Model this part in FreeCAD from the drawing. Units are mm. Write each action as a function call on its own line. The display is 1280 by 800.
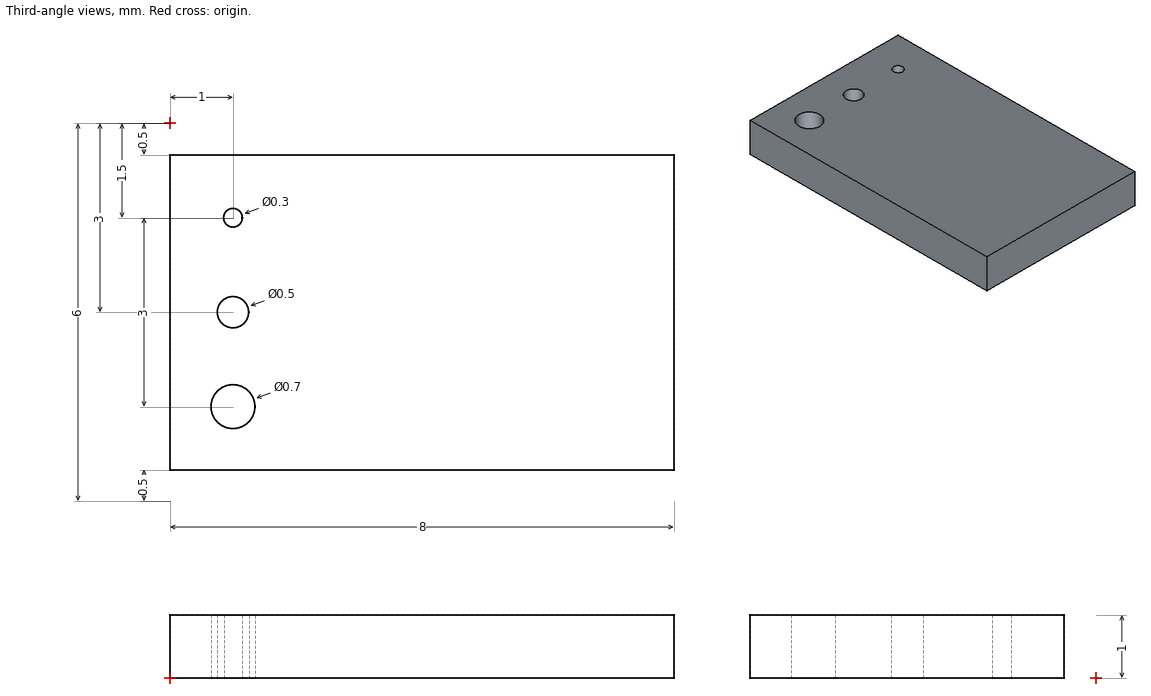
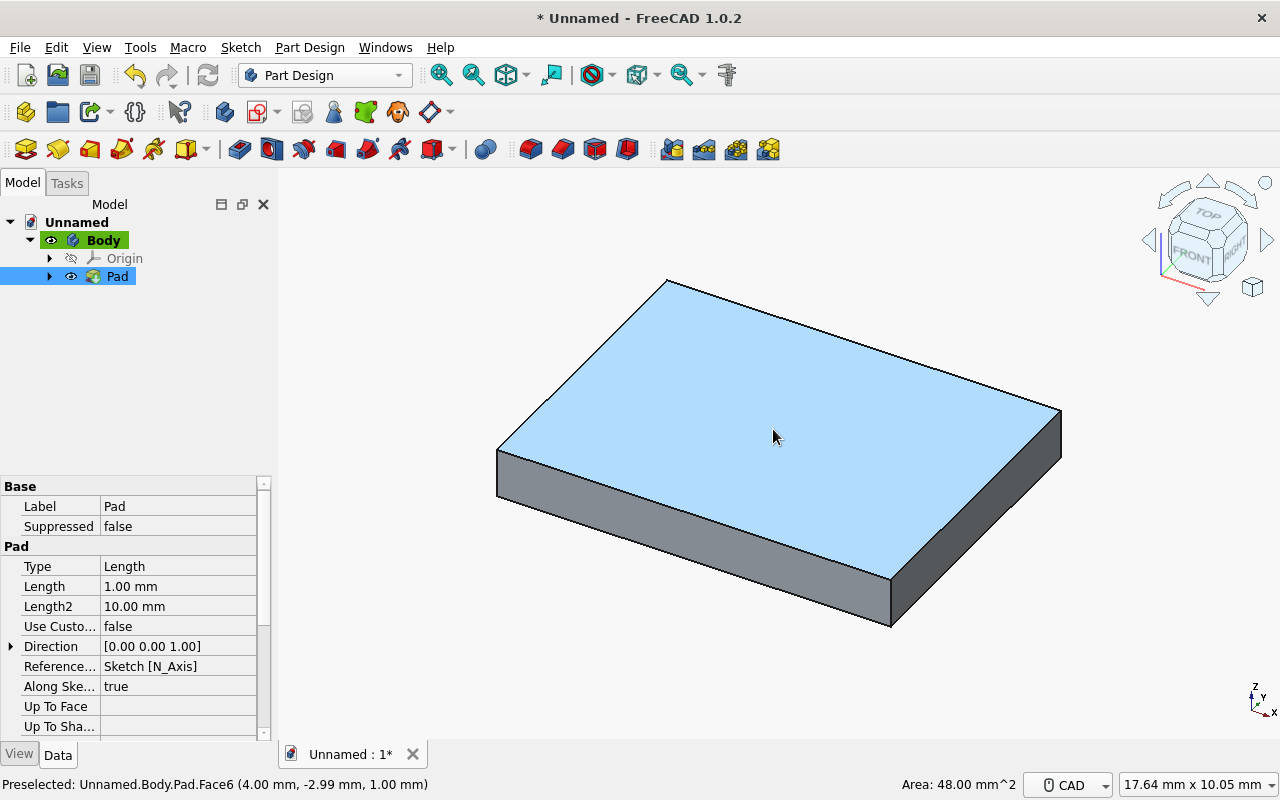
click(258, 112)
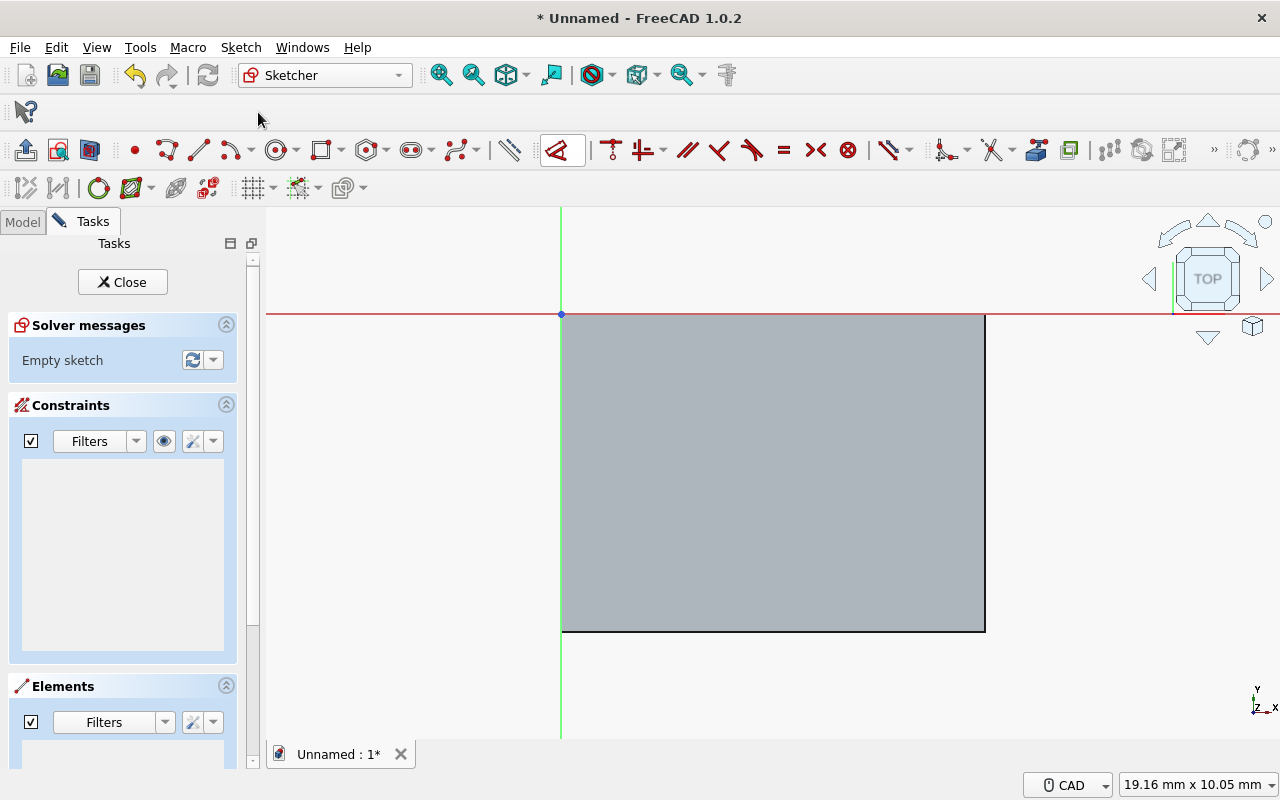
key(g)
key(c)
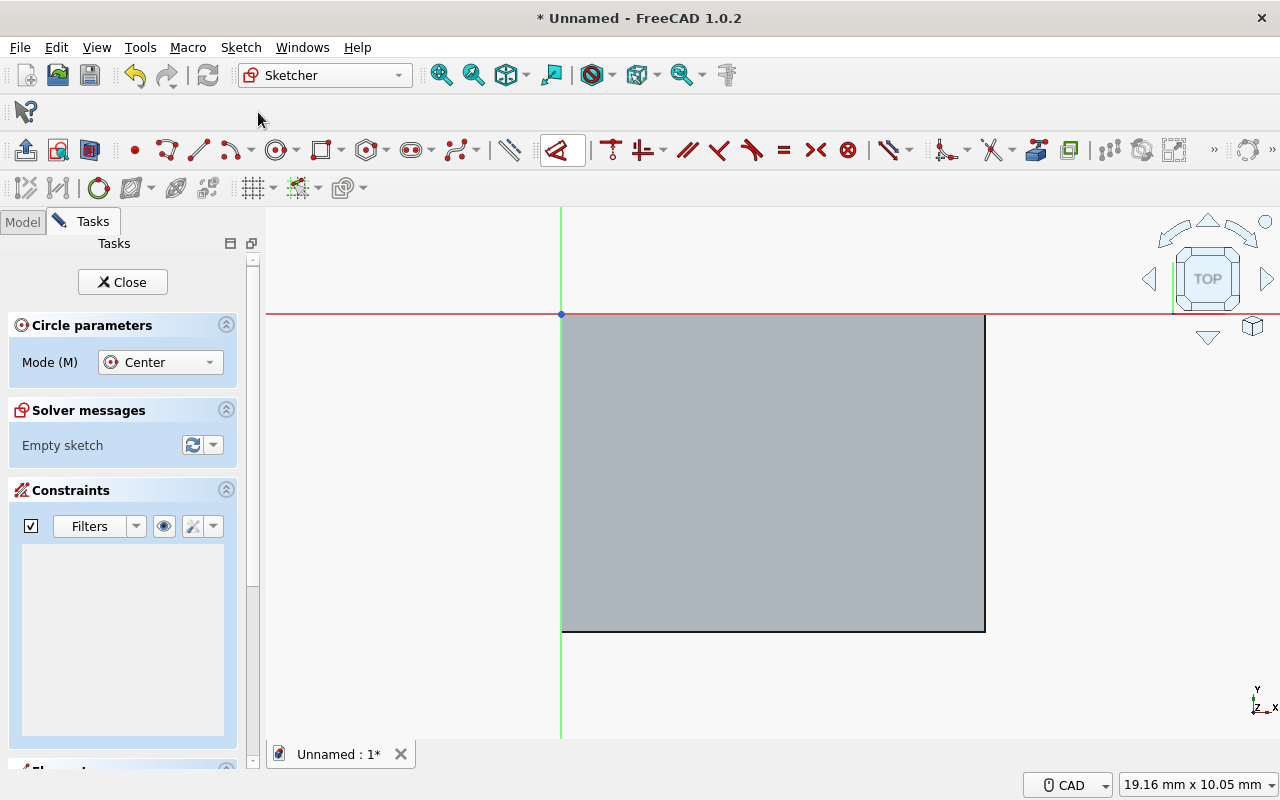
scroll(614, 394, up, 6)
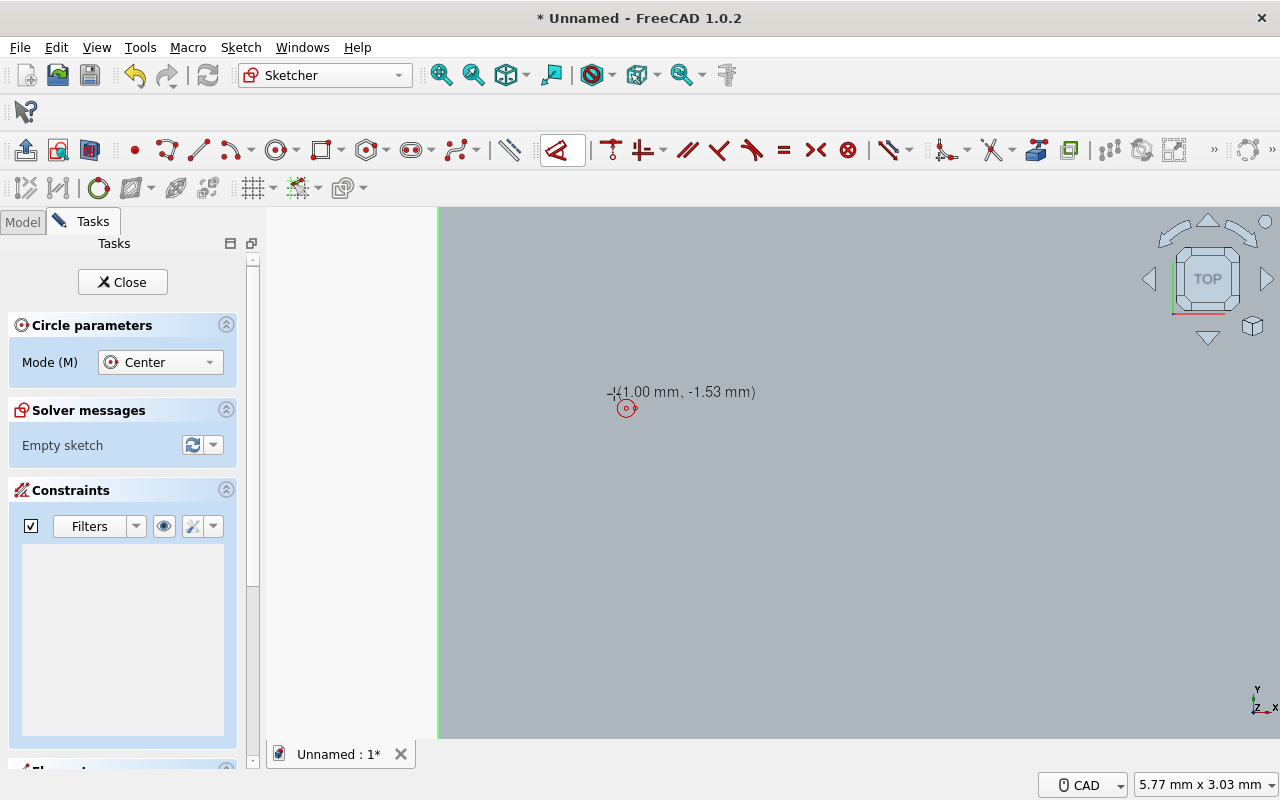
click(614, 392)
click(632, 373)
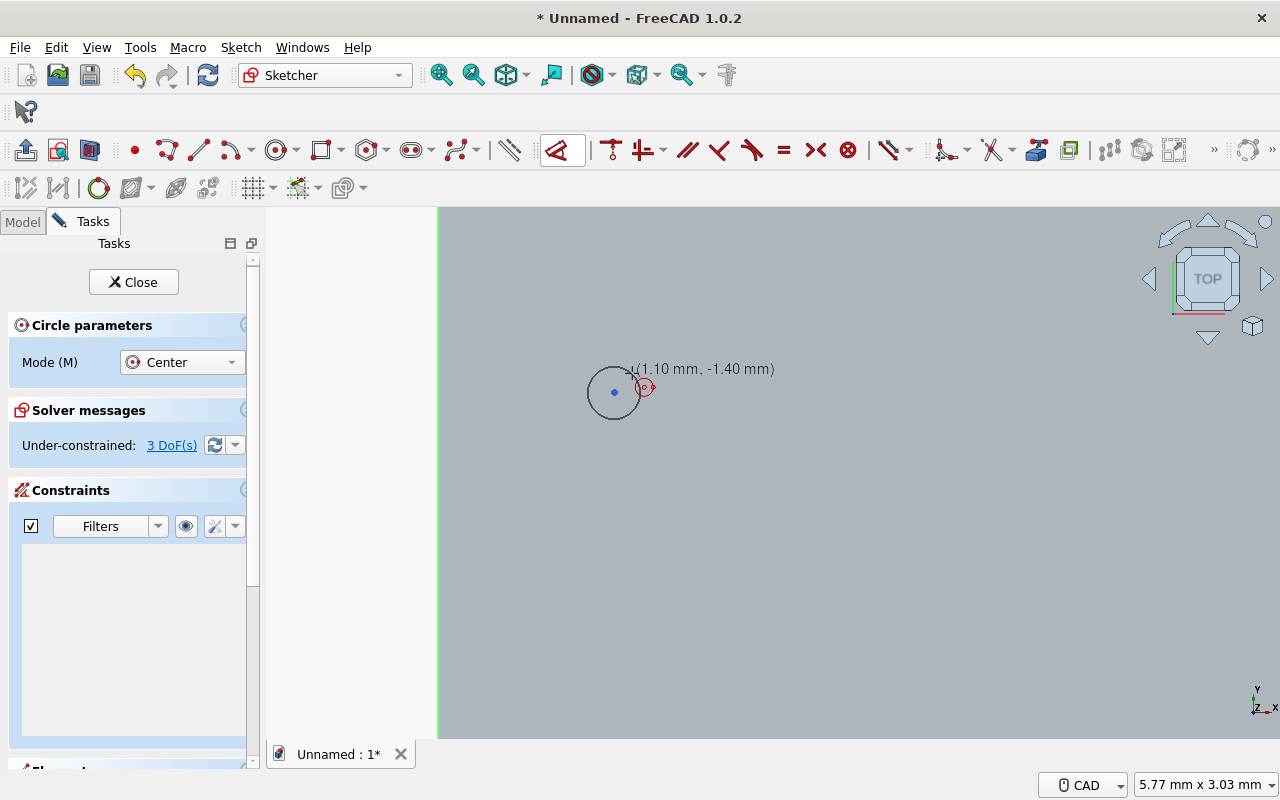
click(614, 655)
click(645, 624)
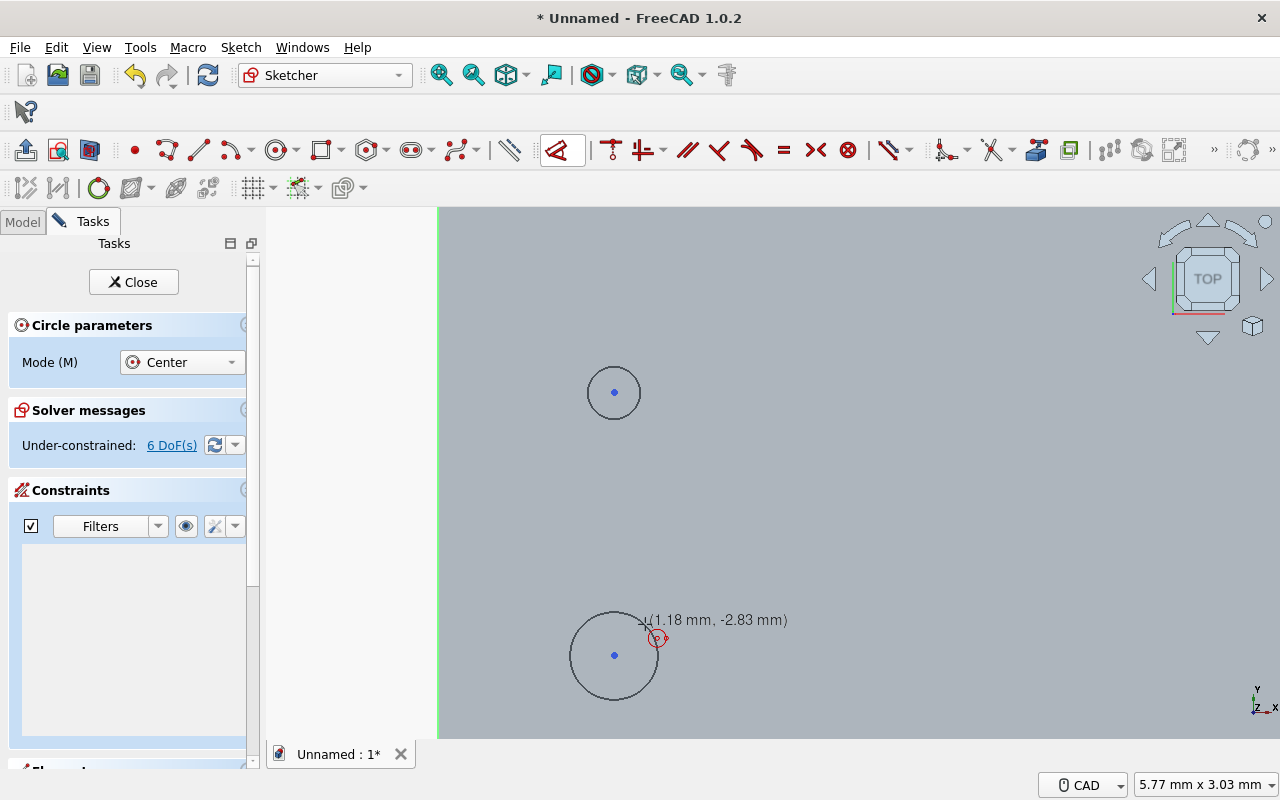
scroll(791, 426, down, 5)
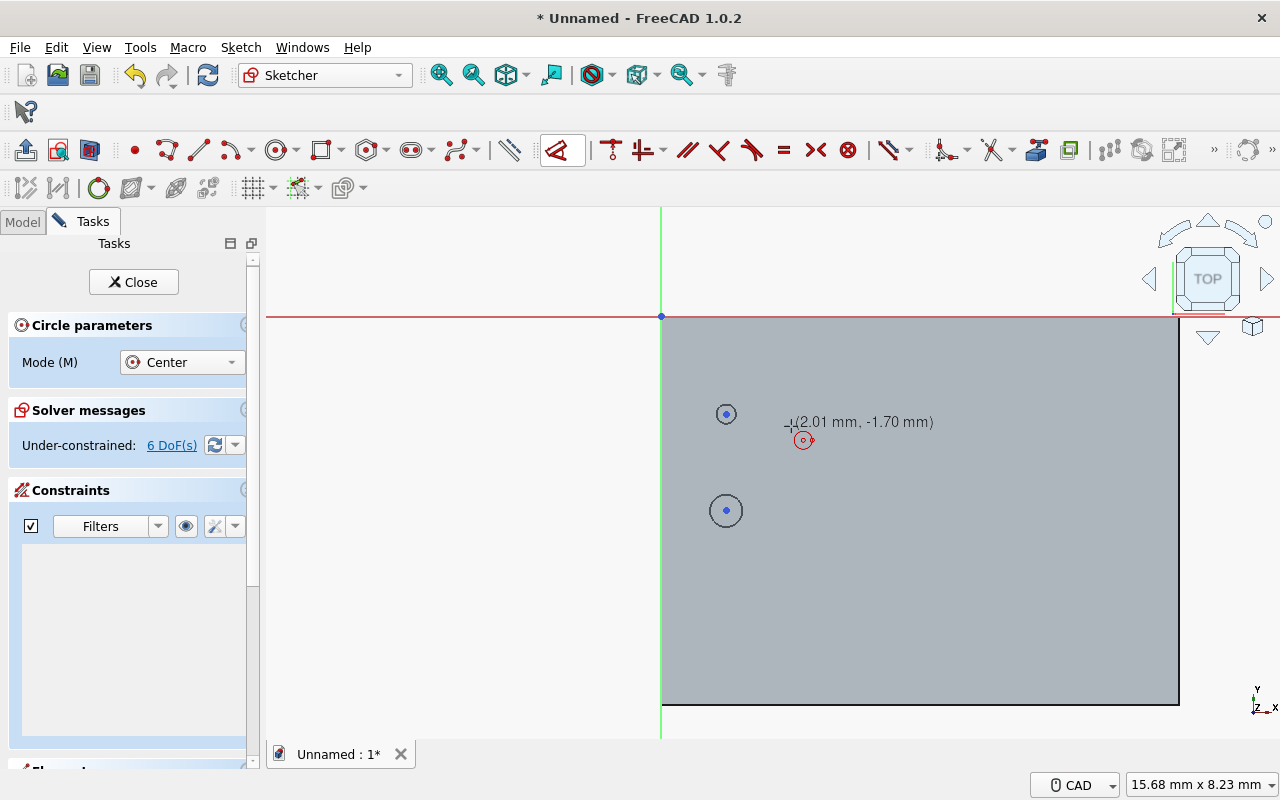
click(726, 608)
click(742, 592)
key(Escape)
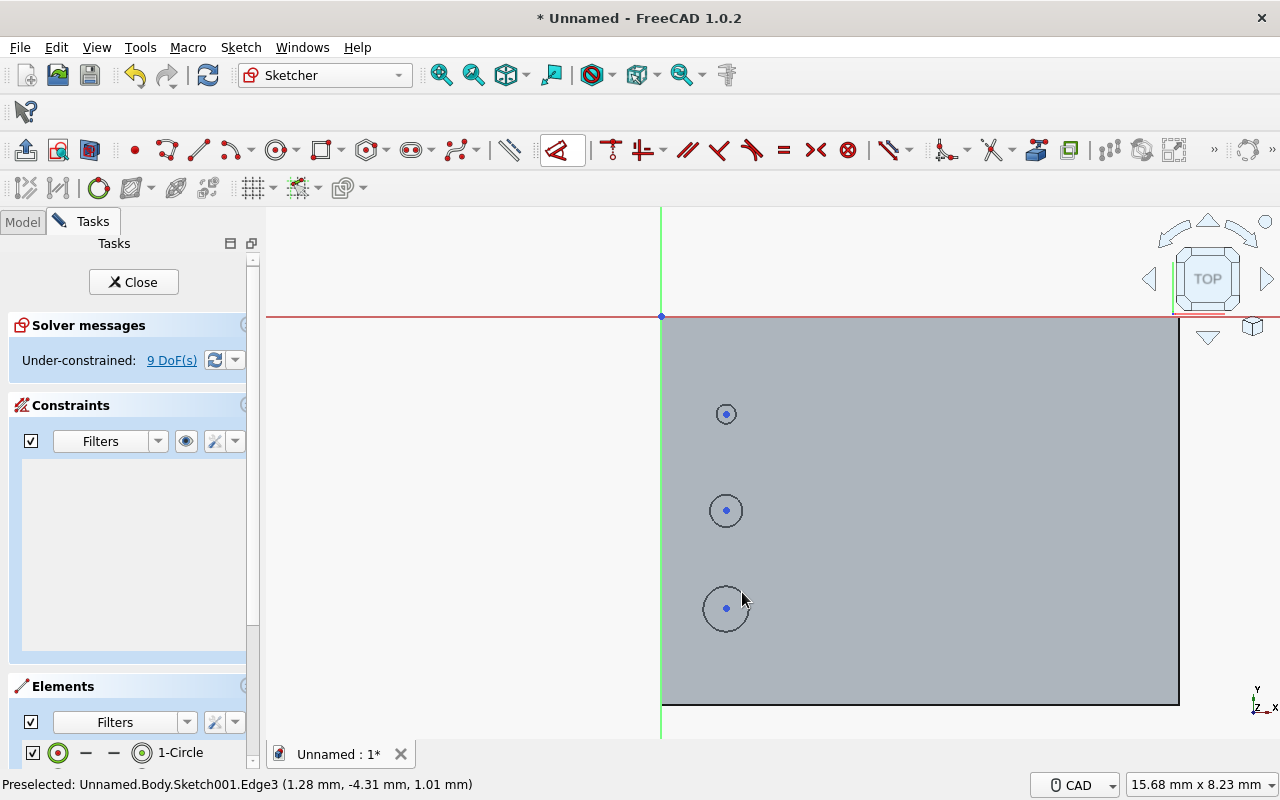
scroll(733, 407, up, 4)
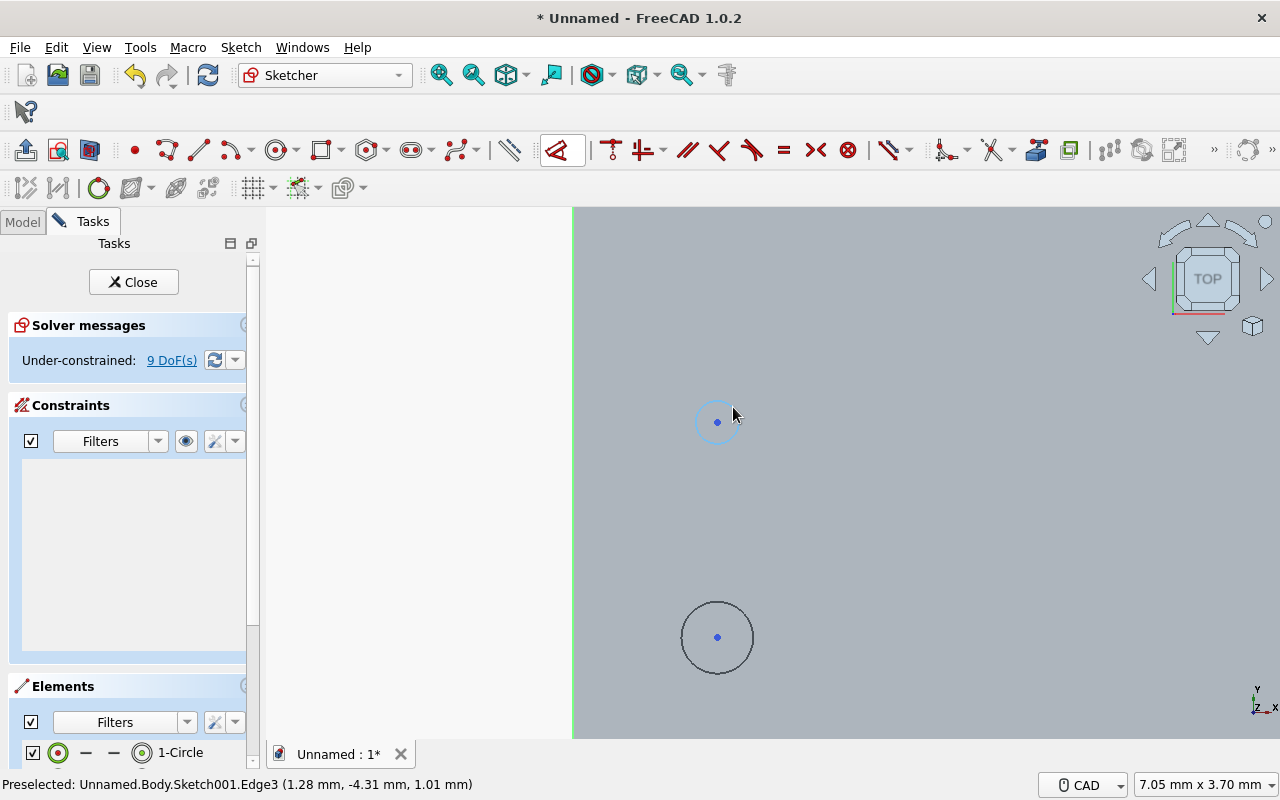
click(732, 407)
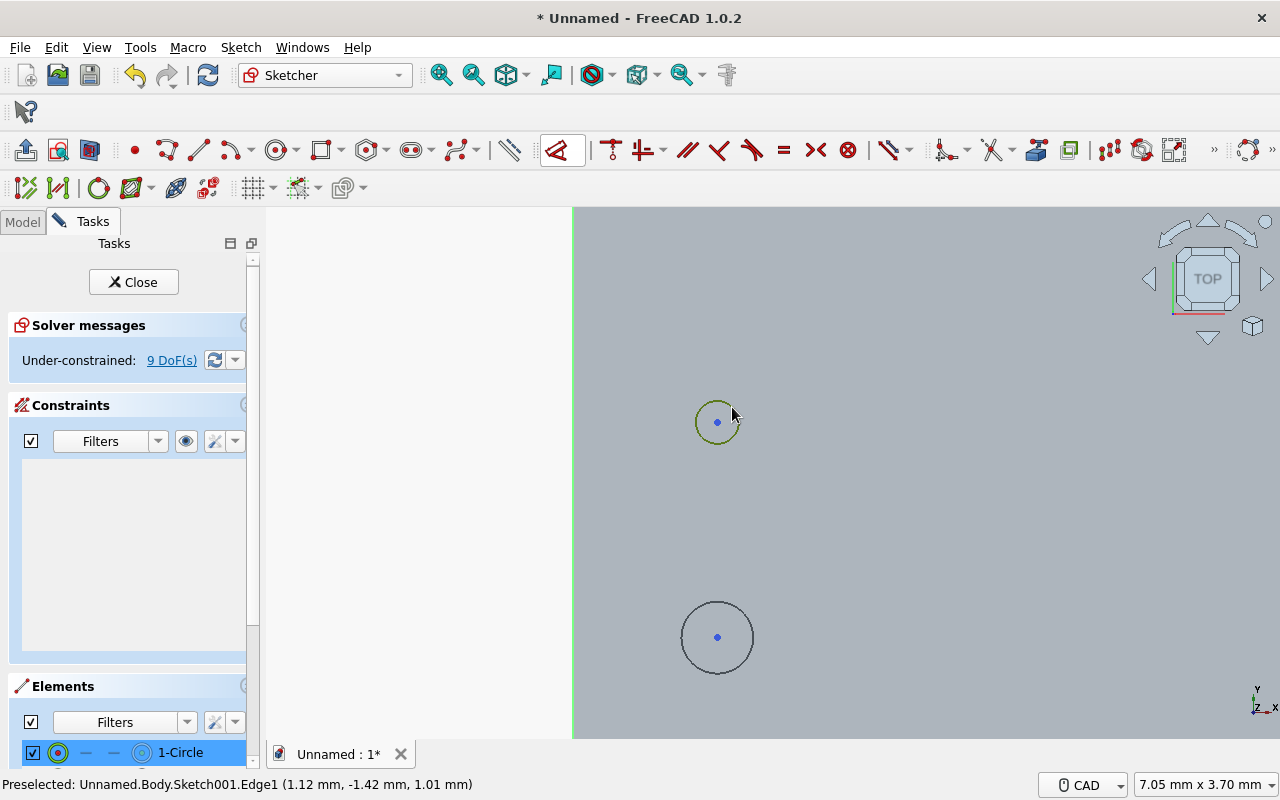
click(580, 150)